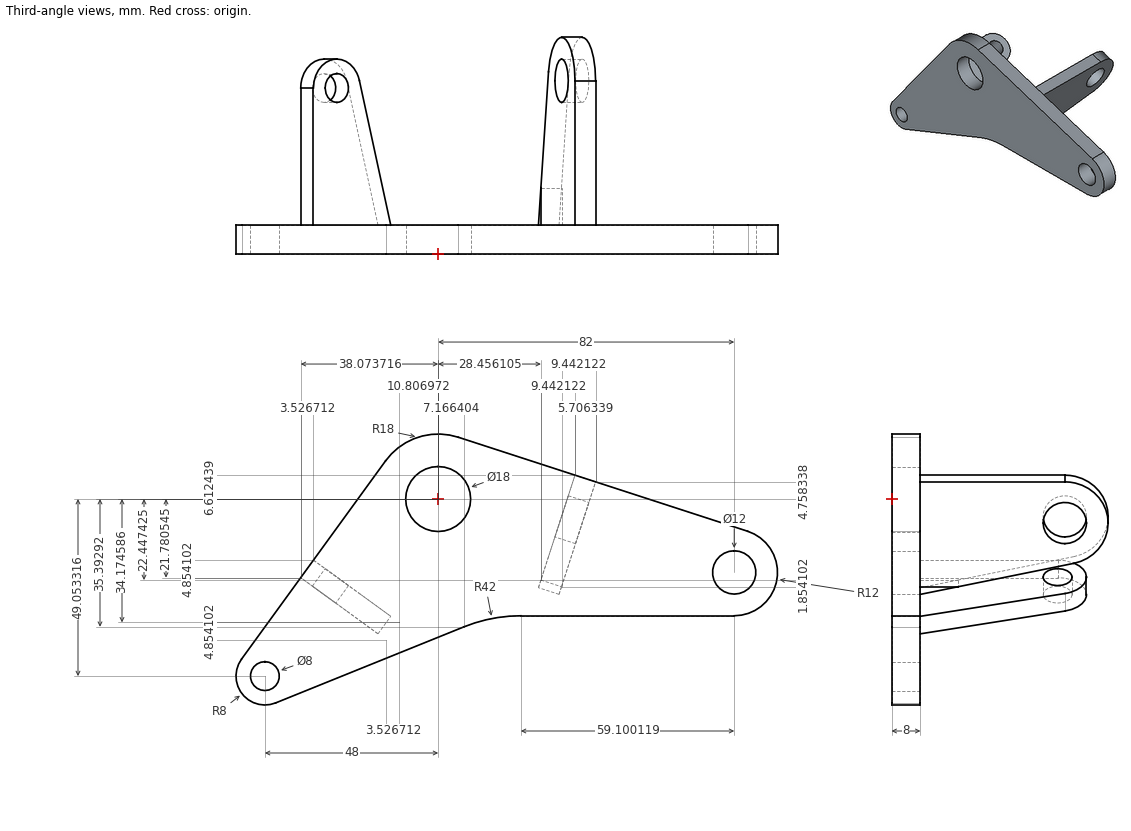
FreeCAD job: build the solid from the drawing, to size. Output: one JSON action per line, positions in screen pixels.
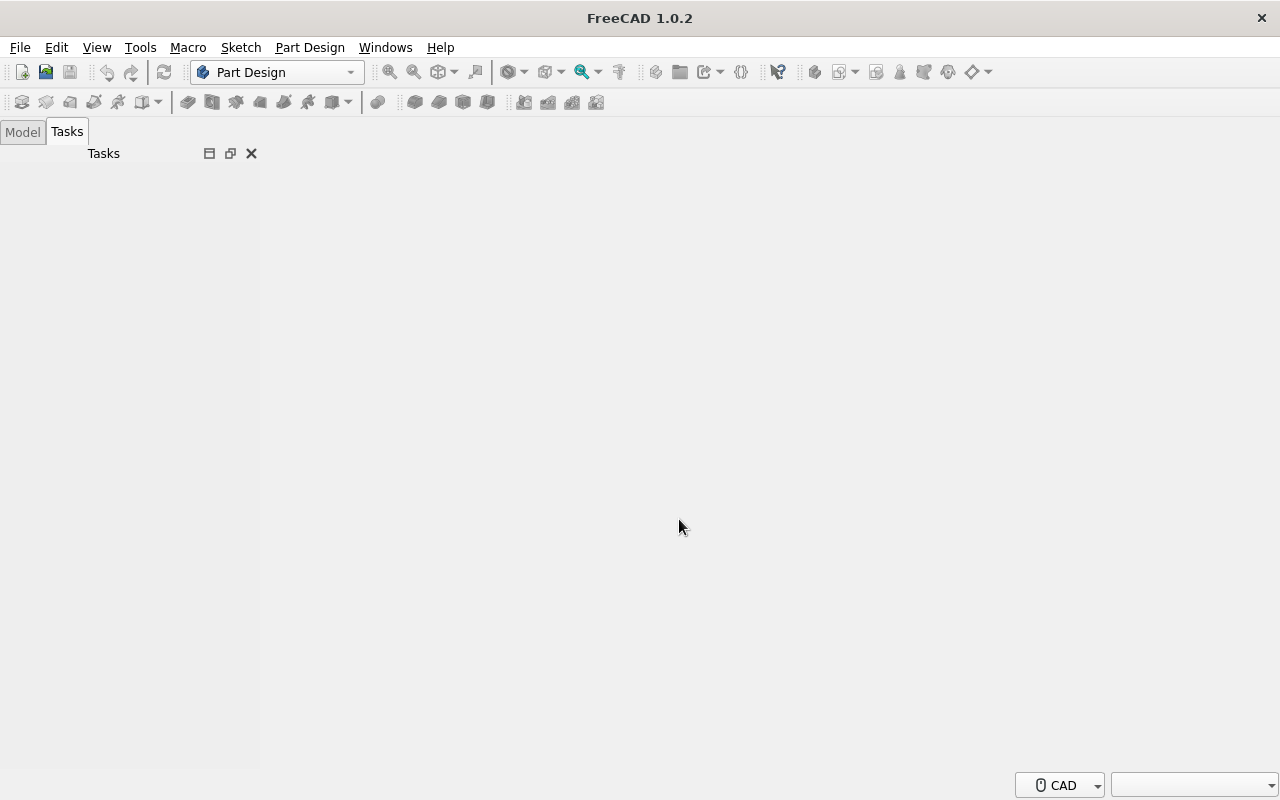
{"action": "left_click", "coordinate": [22, 72]}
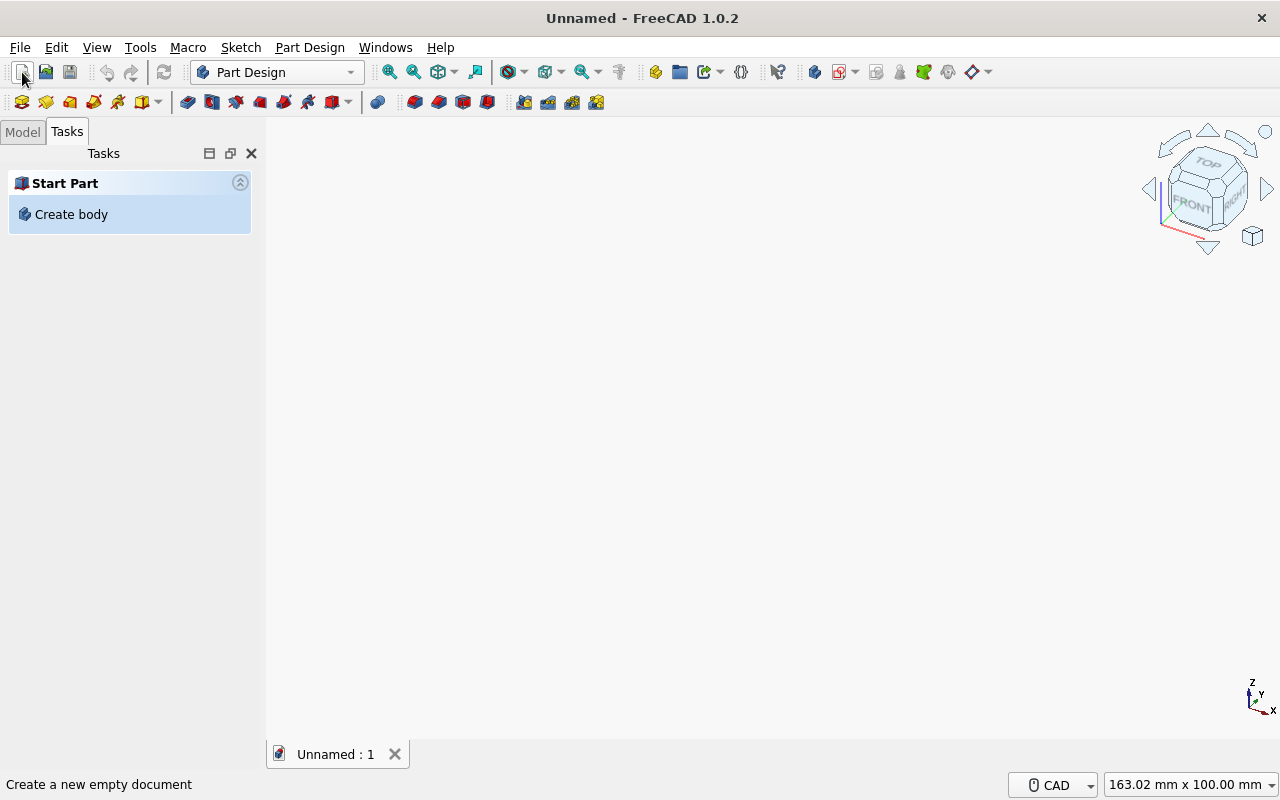
{"action": "left_click", "coordinate": [840, 72]}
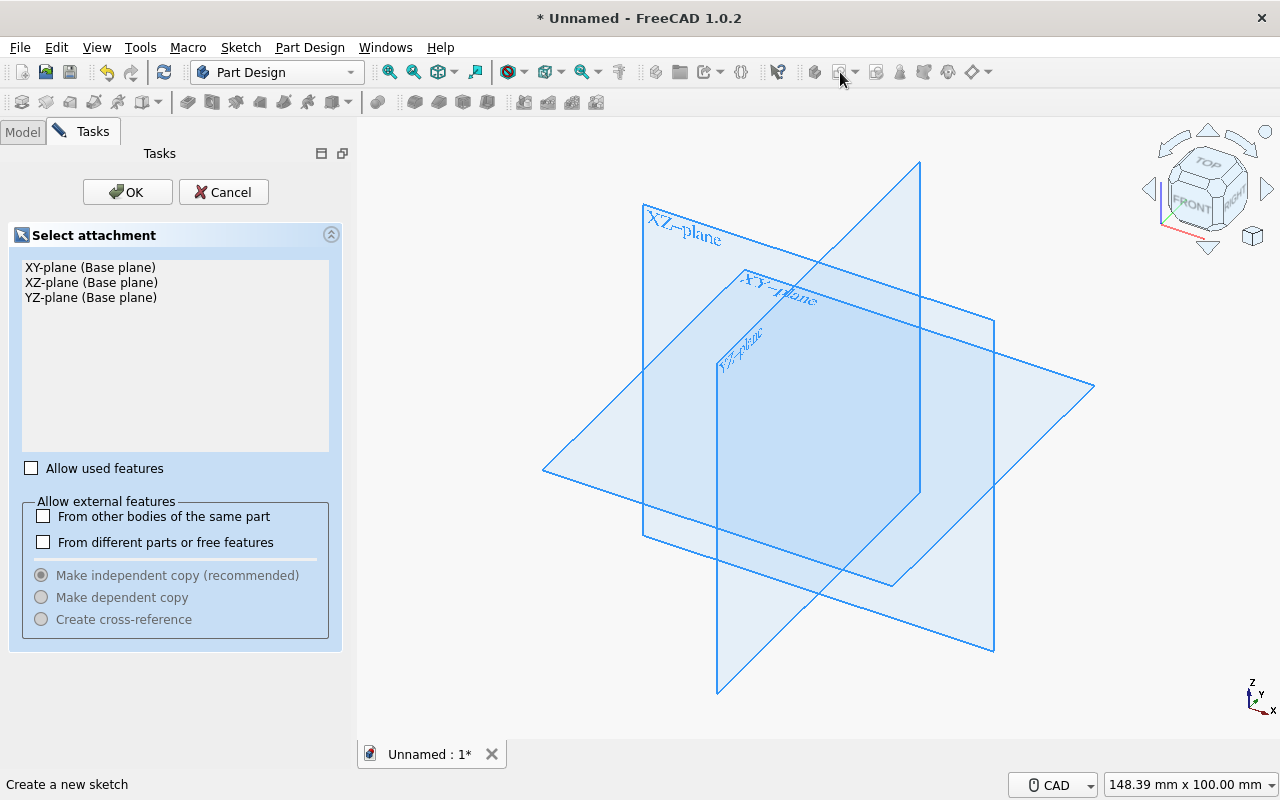
{"action": "left_click", "coordinate": [82, 282]}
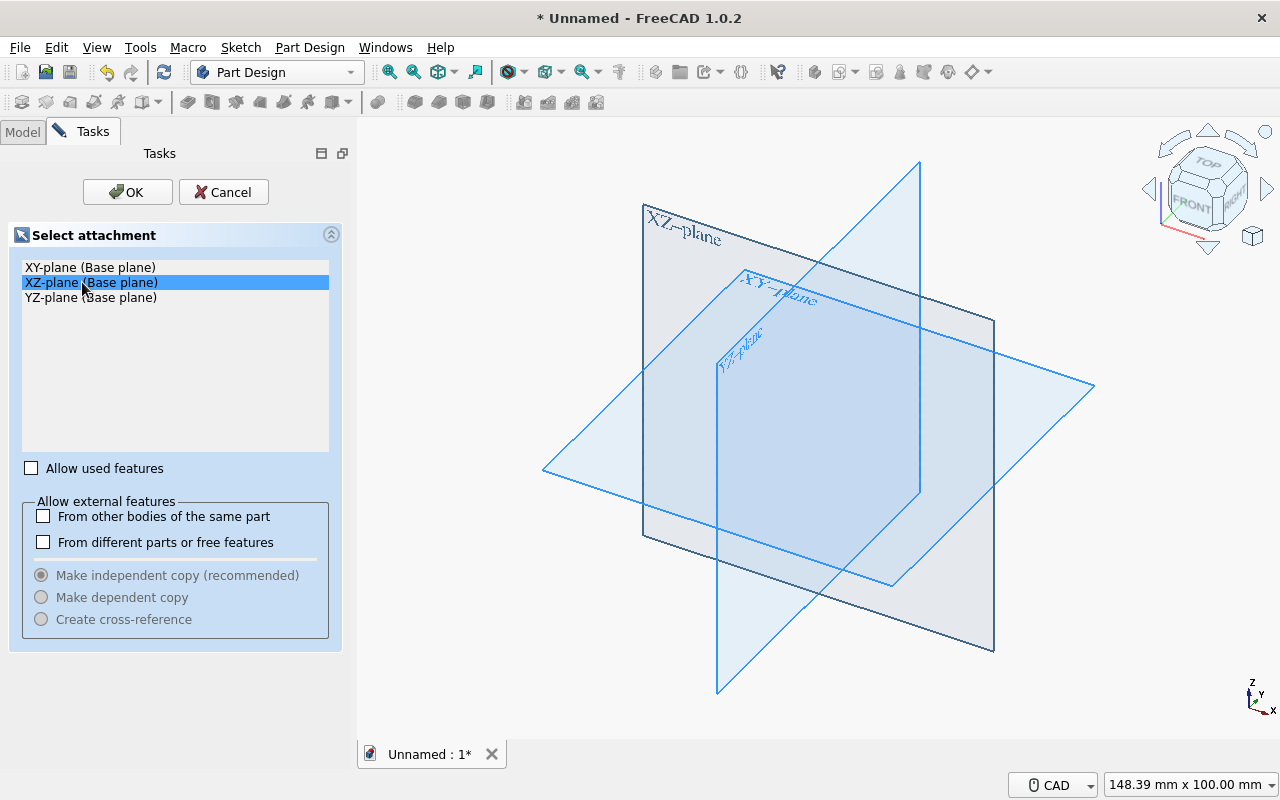
{"action": "left_click", "coordinate": [128, 192]}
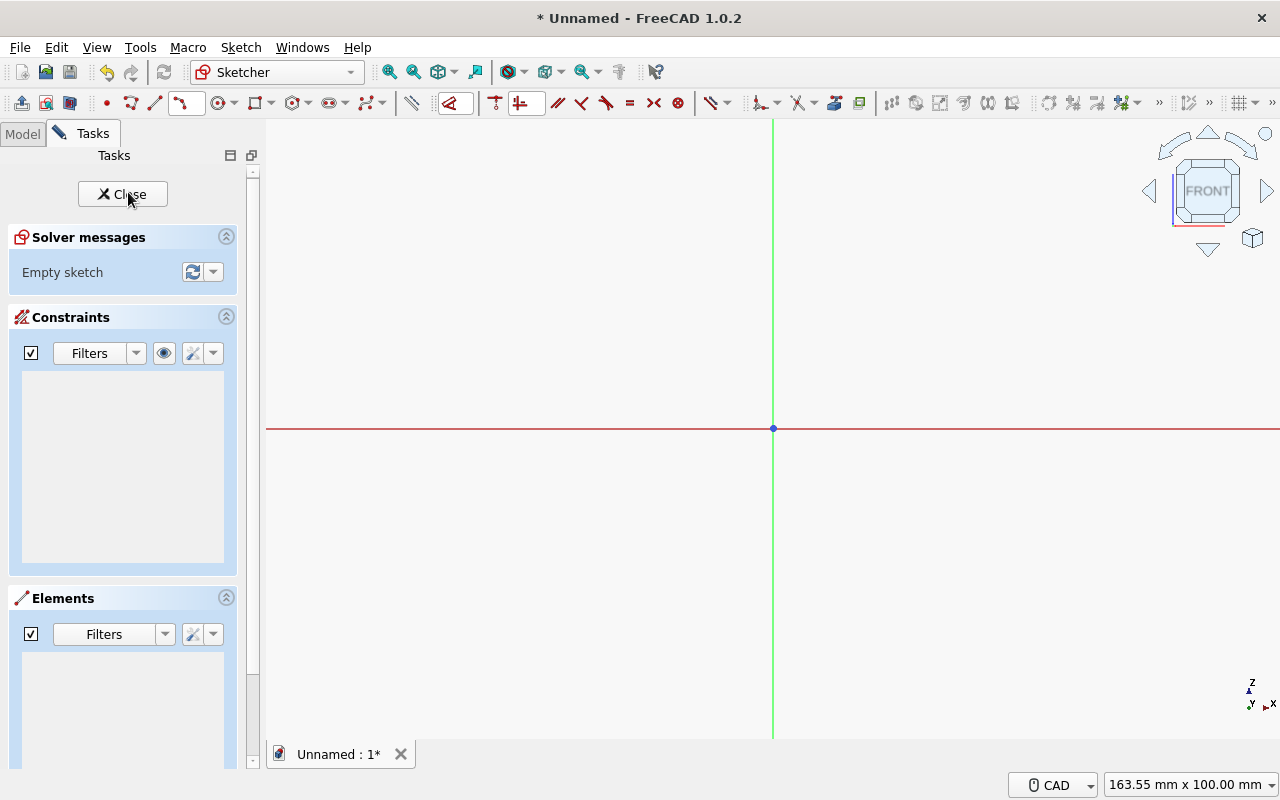
{"action": "scroll", "coordinate": [317, 181], "scroll_direction": "down", "scroll_amount": 2}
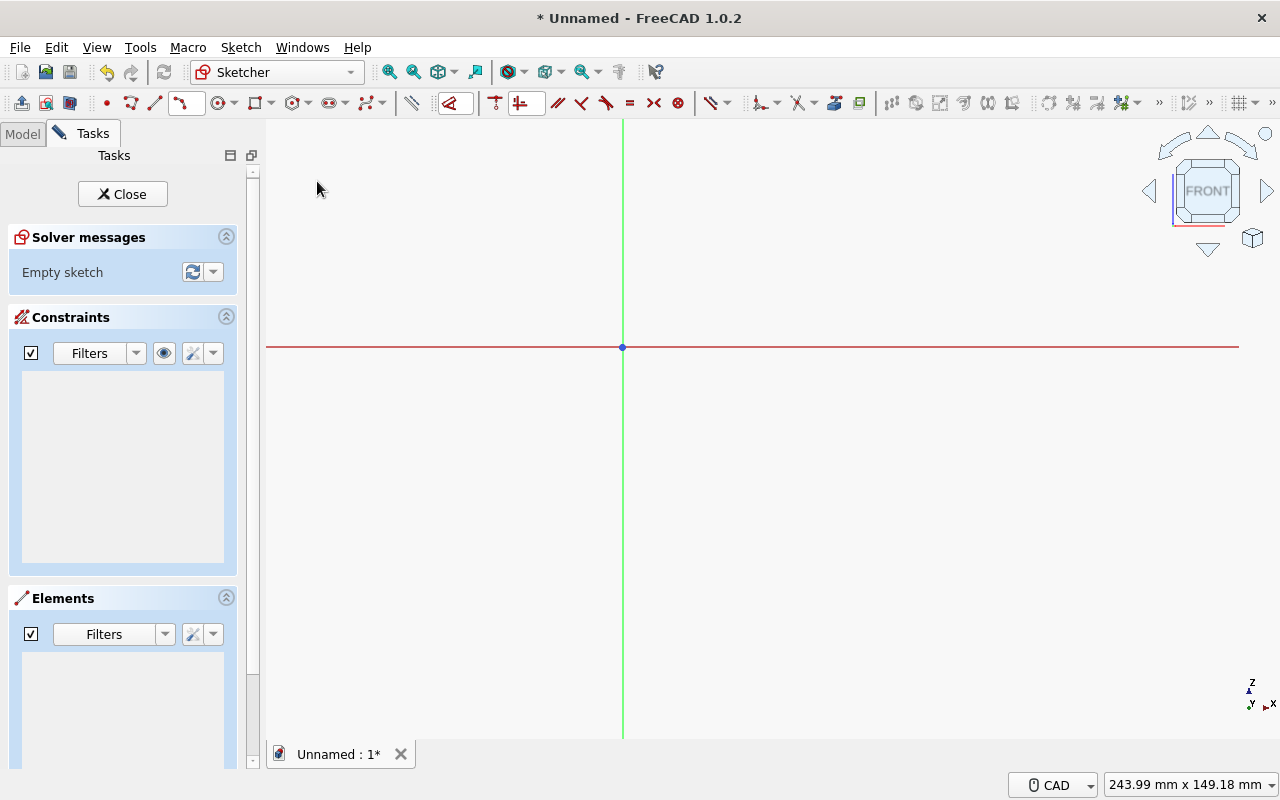
{"action": "left_click", "coordinate": [156, 104]}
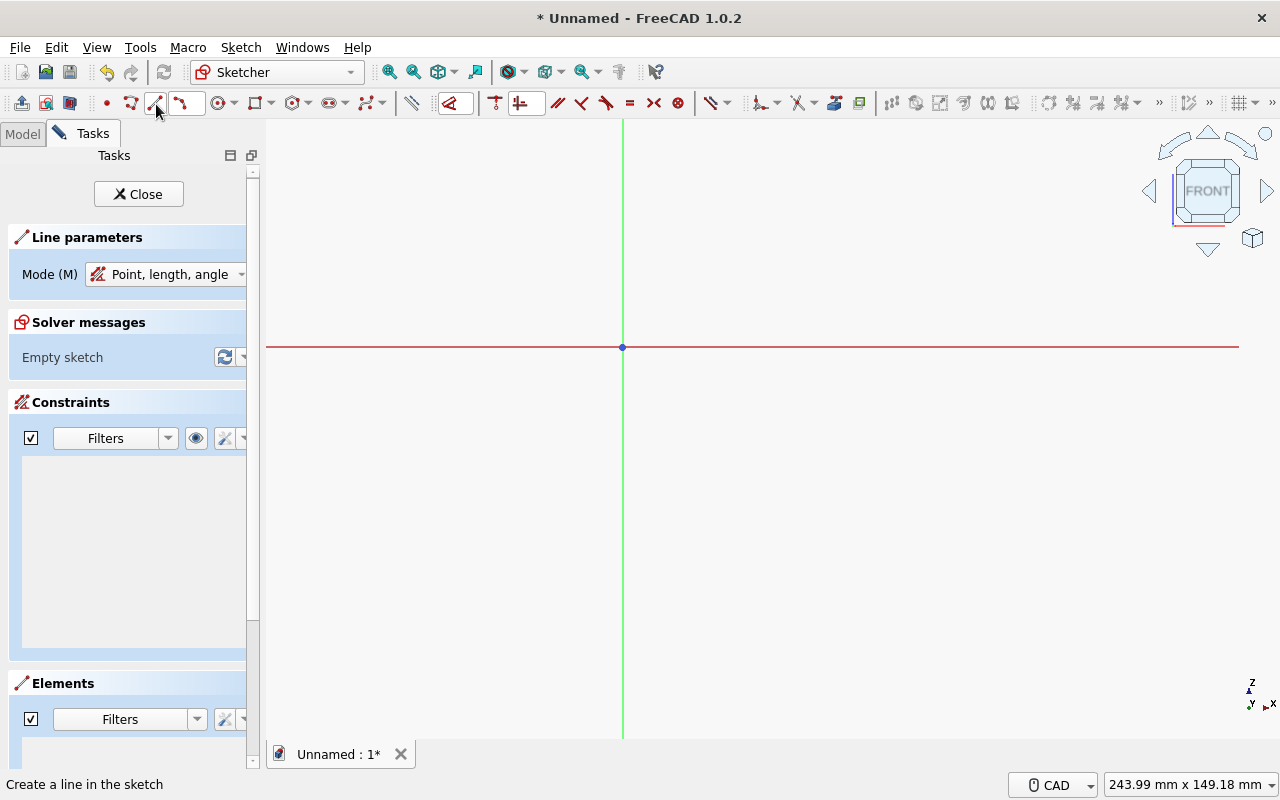
{"action": "left_click", "coordinate": [963, 482]}
{"action": "left_click", "coordinate": [718, 482]}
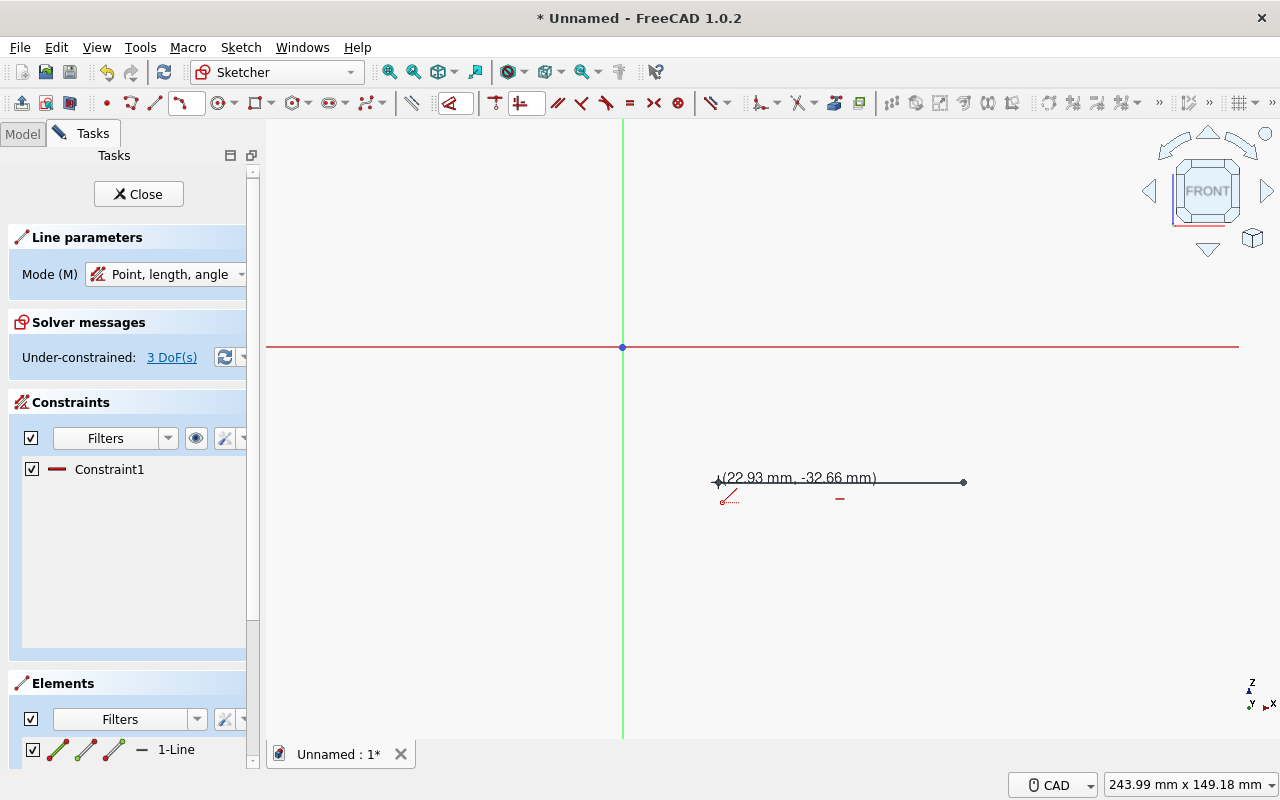
{"action": "left_click", "coordinate": [652, 494]}
{"action": "left_click", "coordinate": [436, 582]}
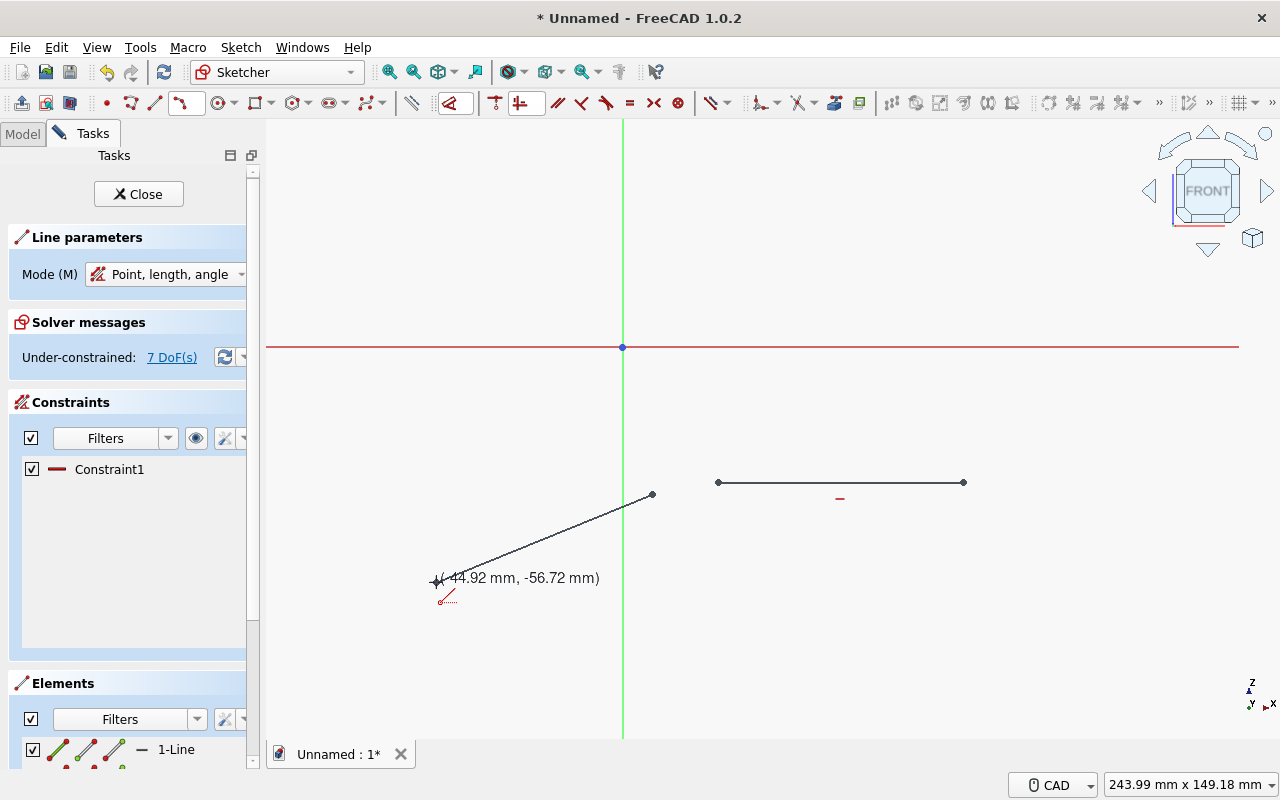
{"action": "left_click", "coordinate": [396, 532]}
{"action": "left_click", "coordinate": [562, 303]}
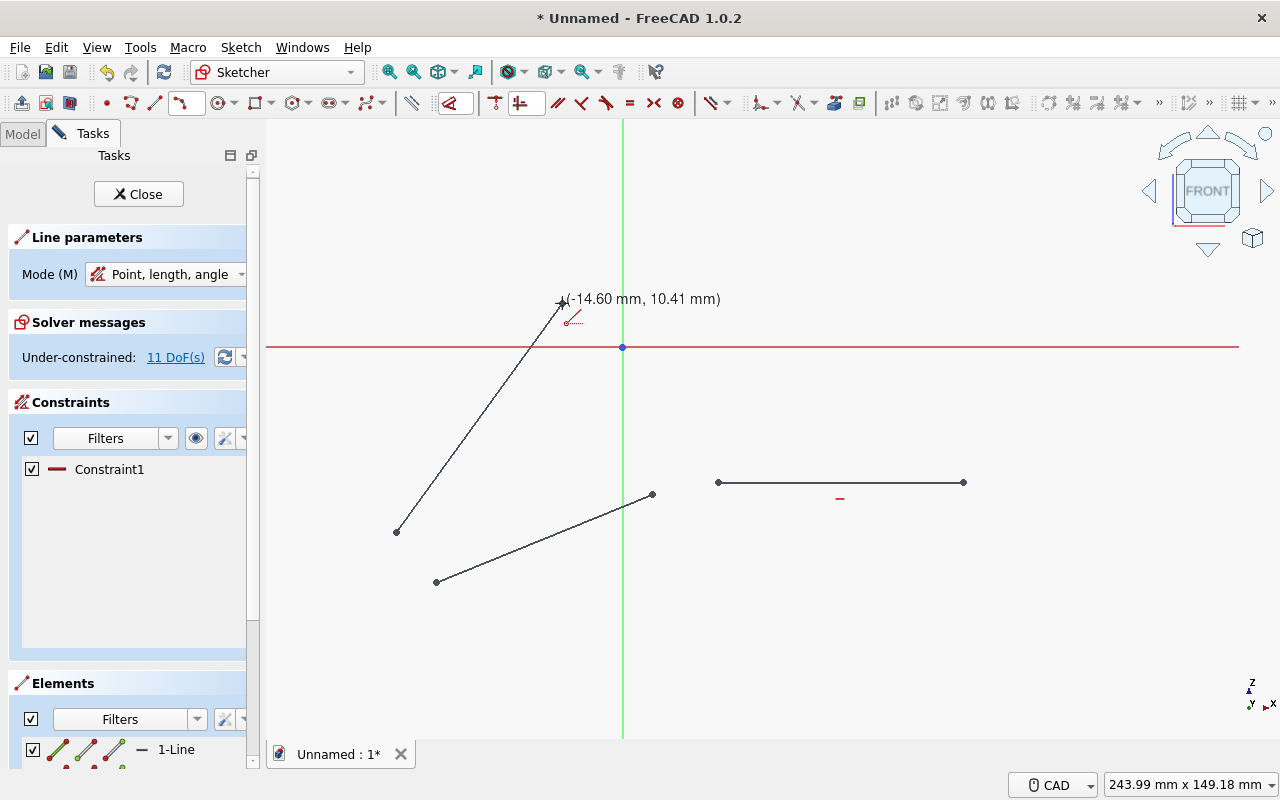
{"action": "left_click", "coordinate": [646, 276]}
{"action": "left_click", "coordinate": [979, 384]}